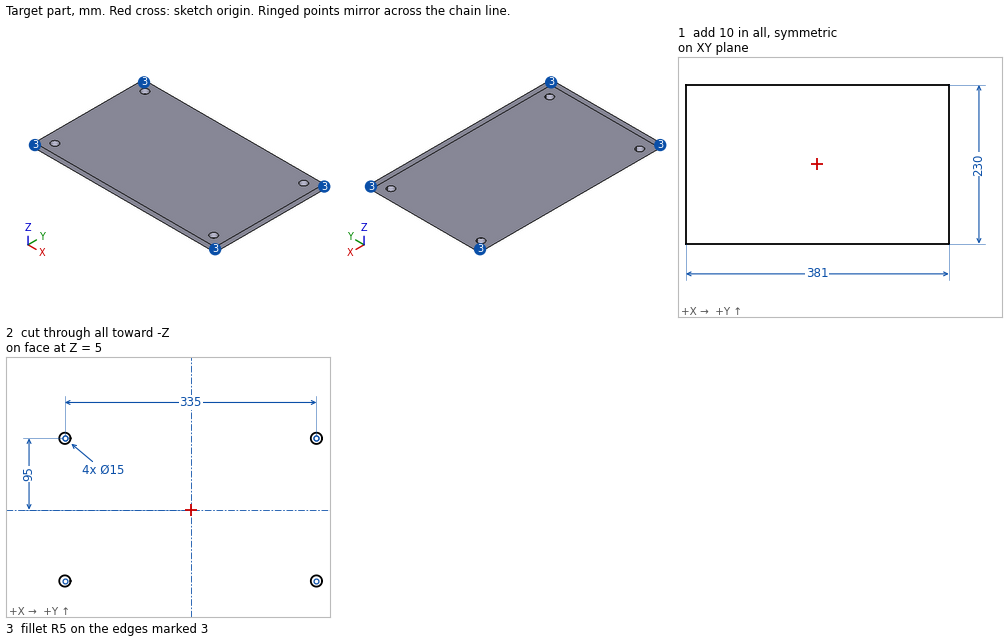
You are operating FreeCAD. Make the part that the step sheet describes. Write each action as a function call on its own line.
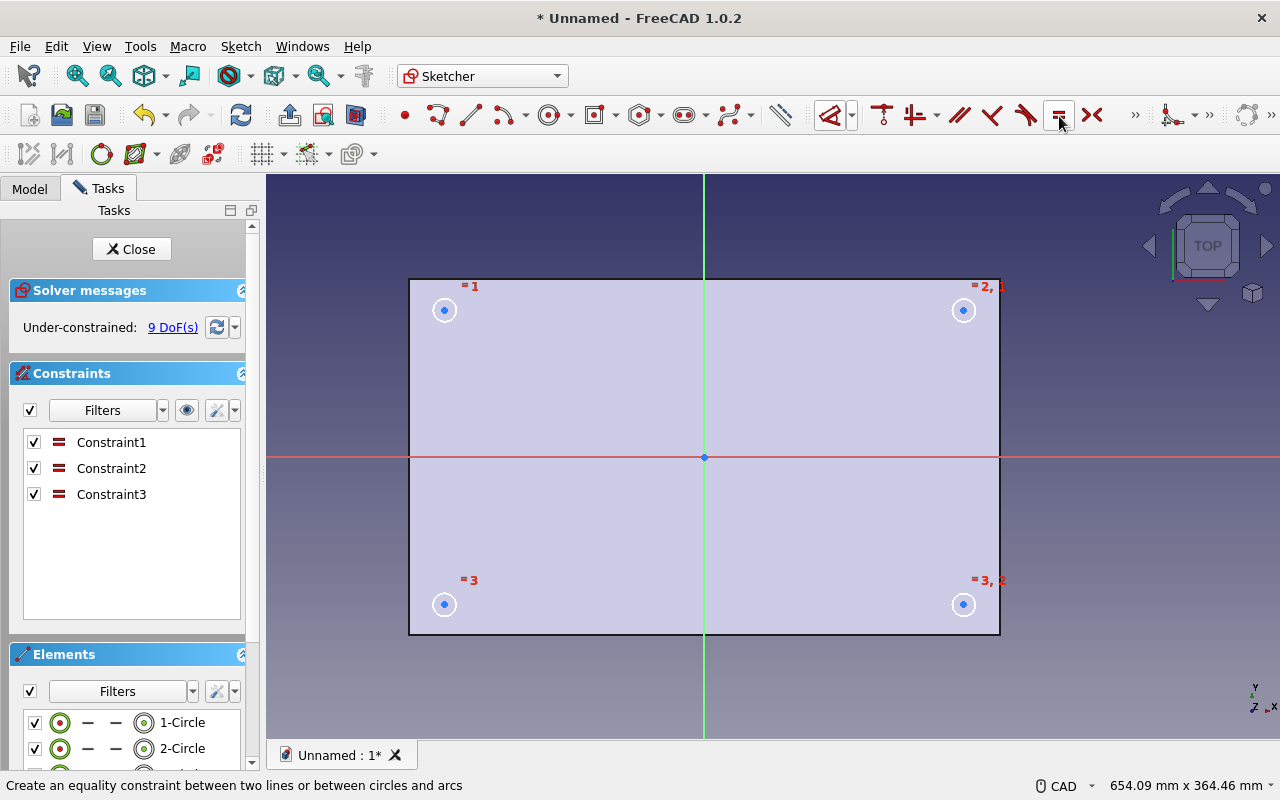
click(445, 310)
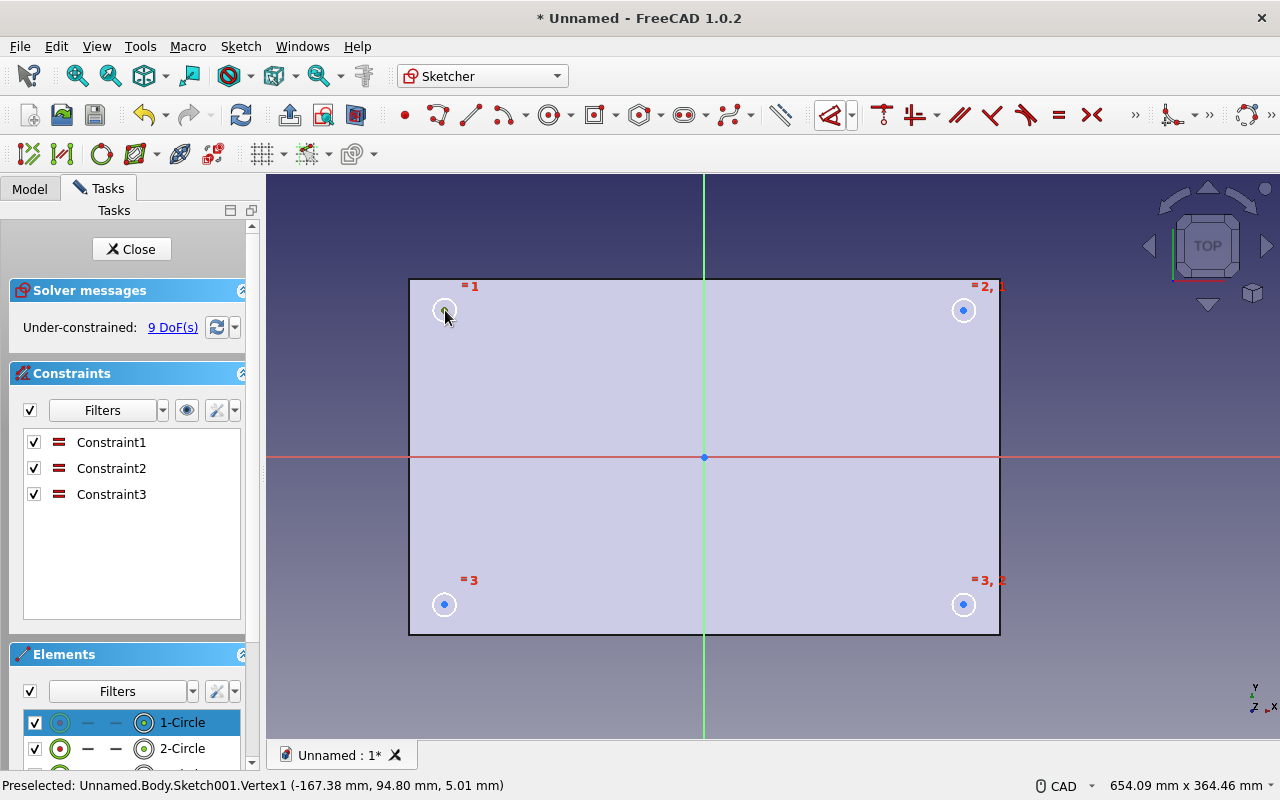
click(964, 311)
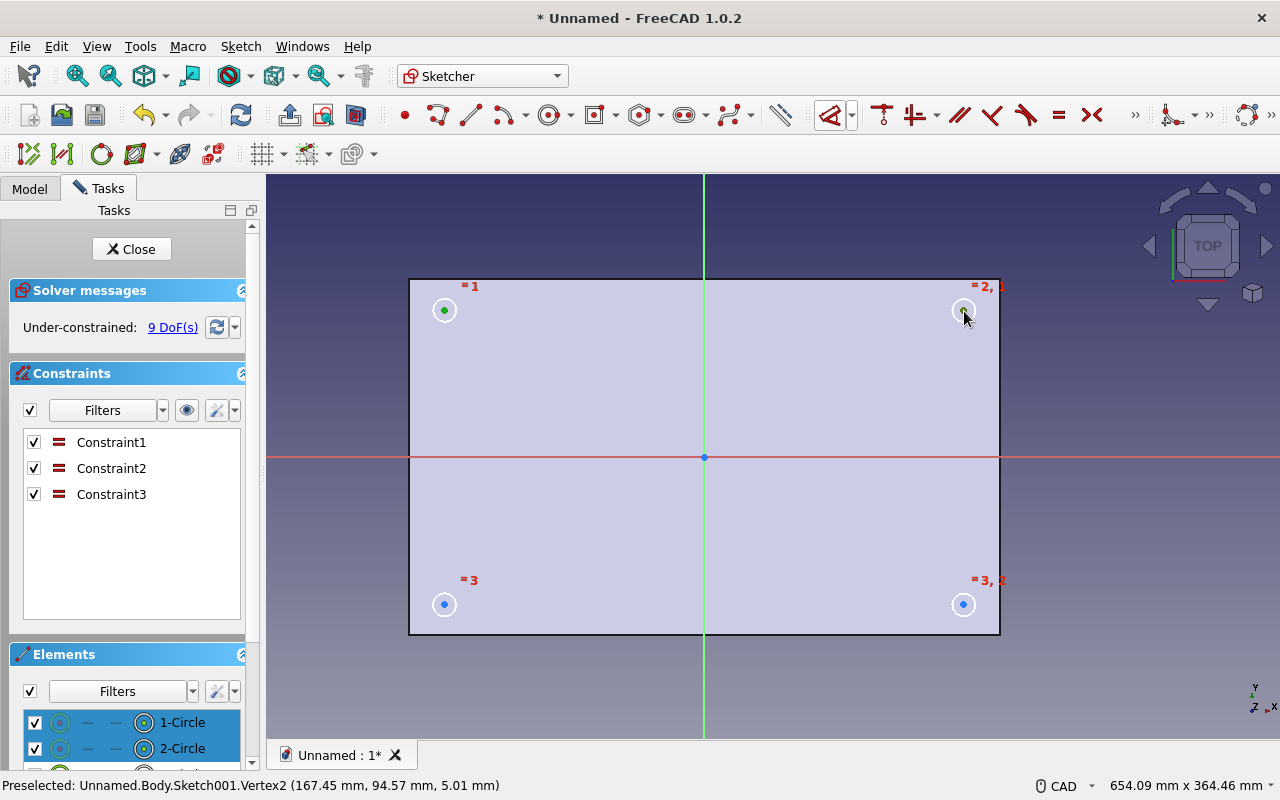
click(704, 675)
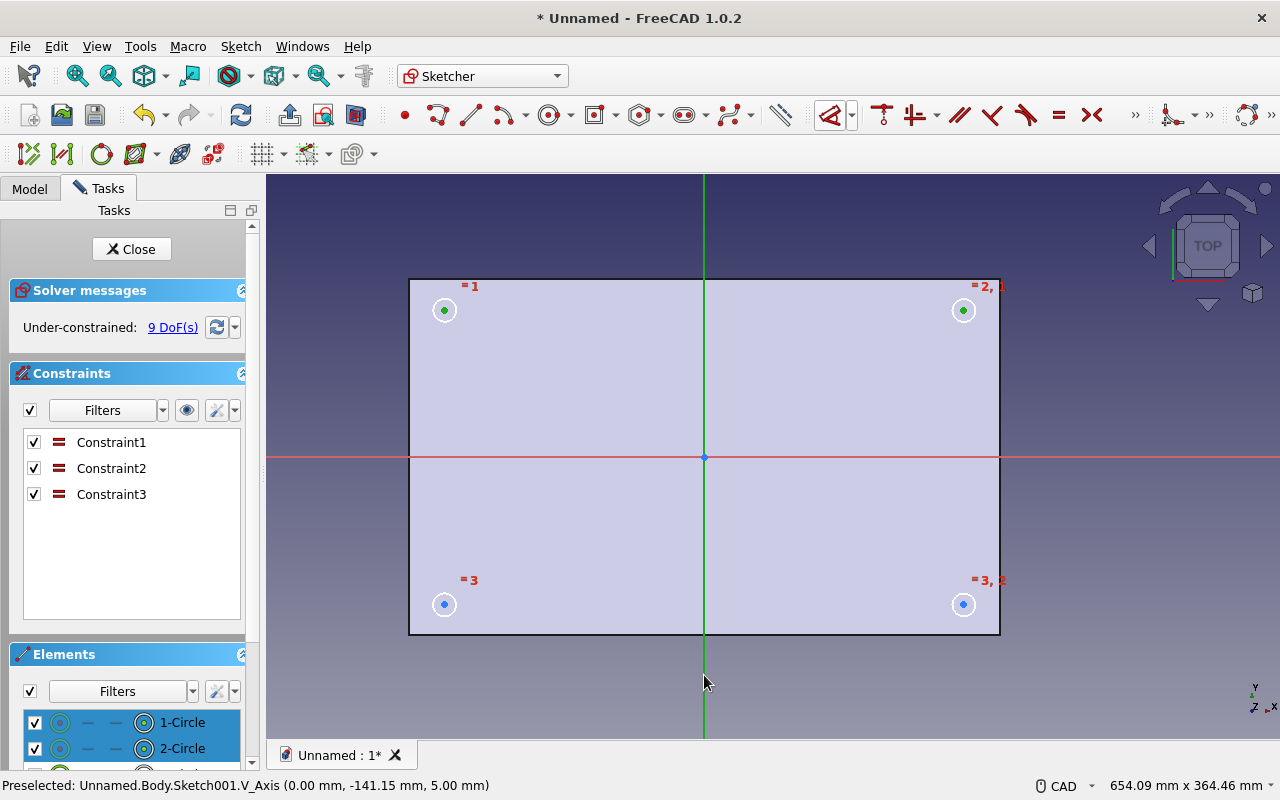
click(1092, 116)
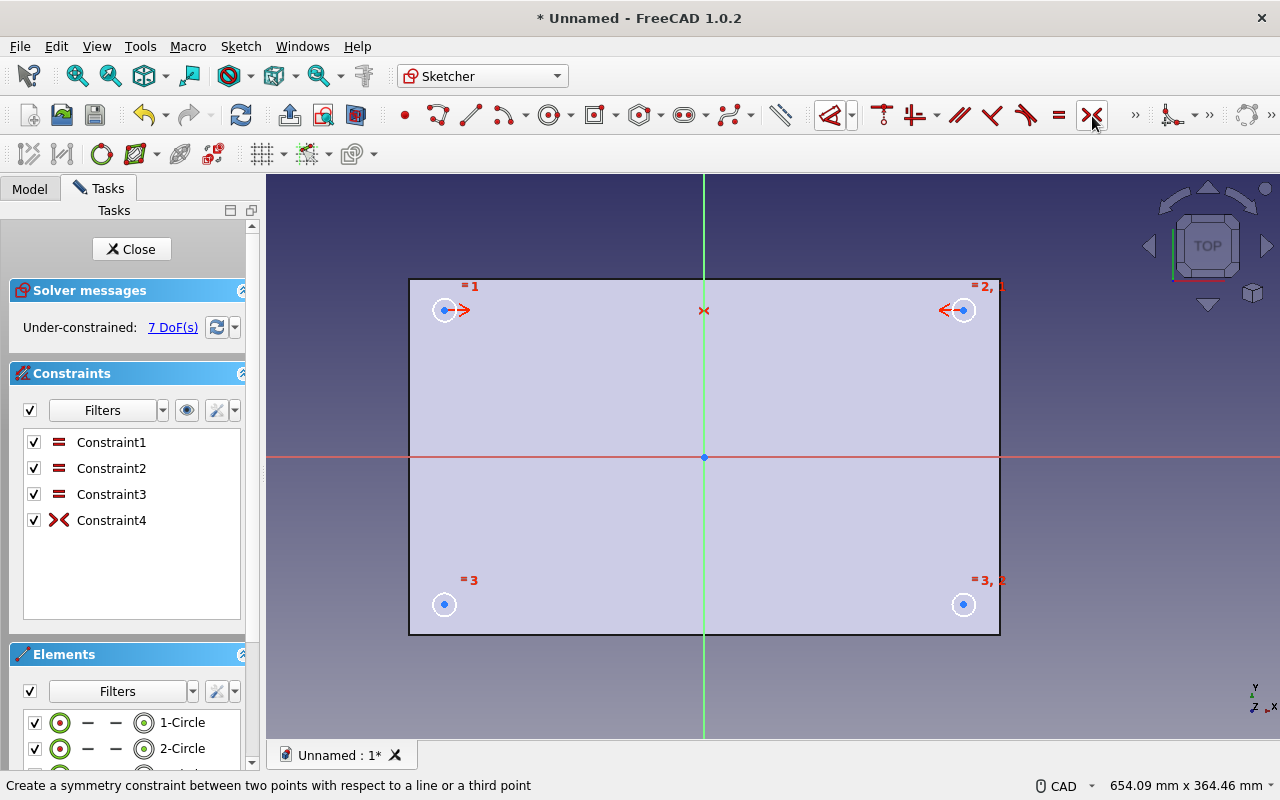
click(964, 310)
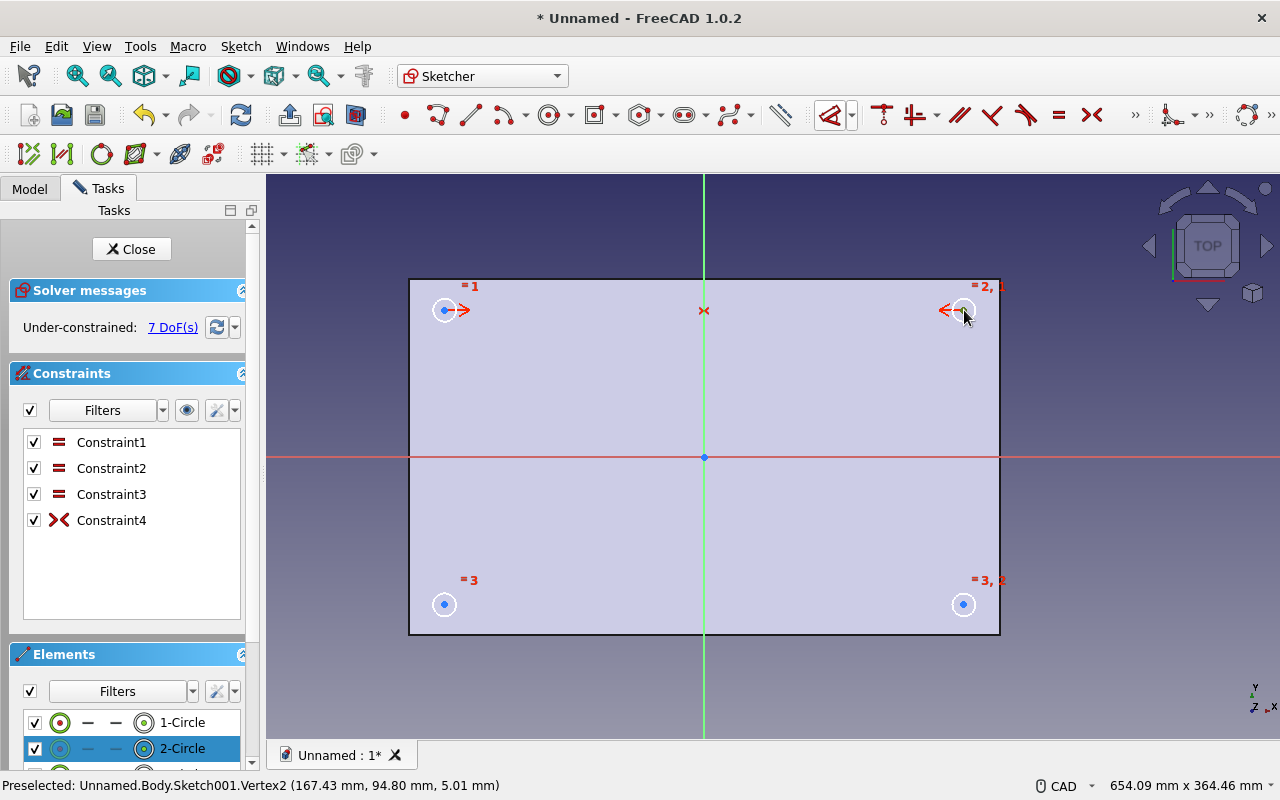
click(964, 605)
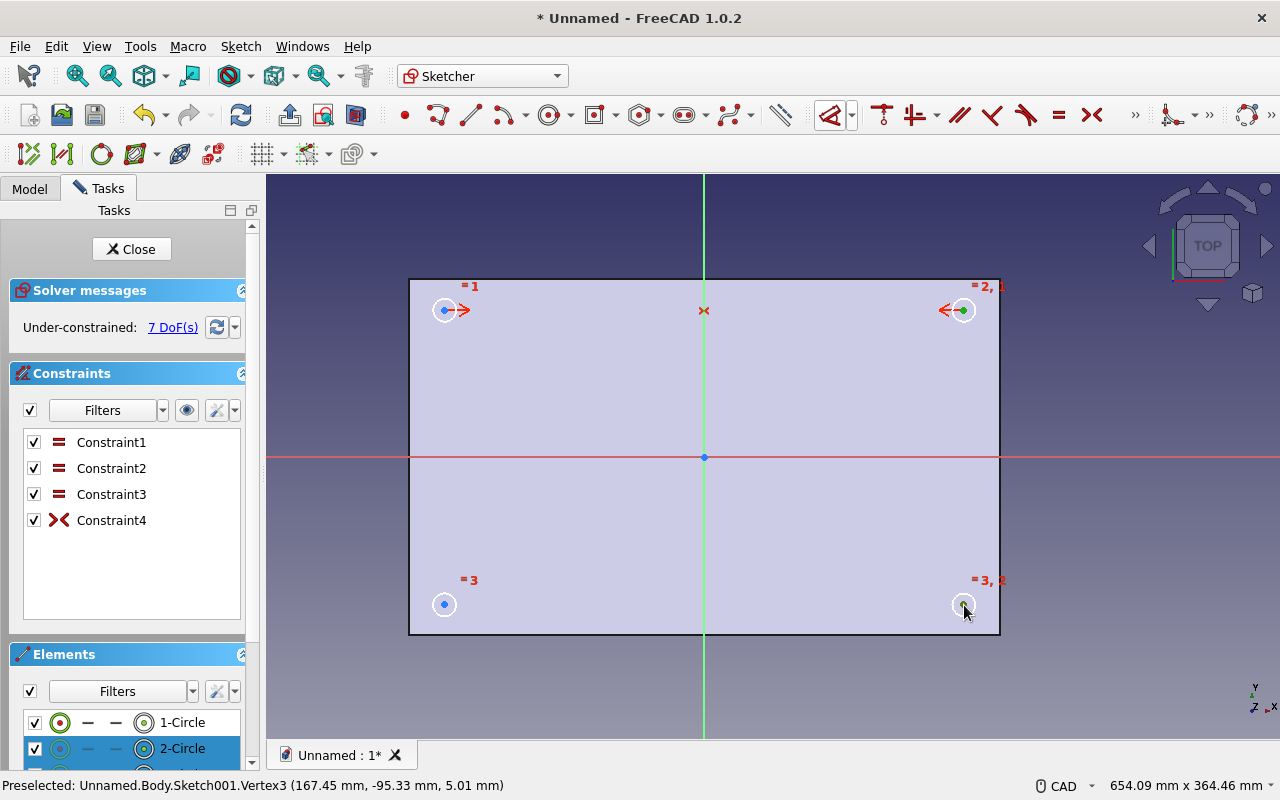
click(353, 457)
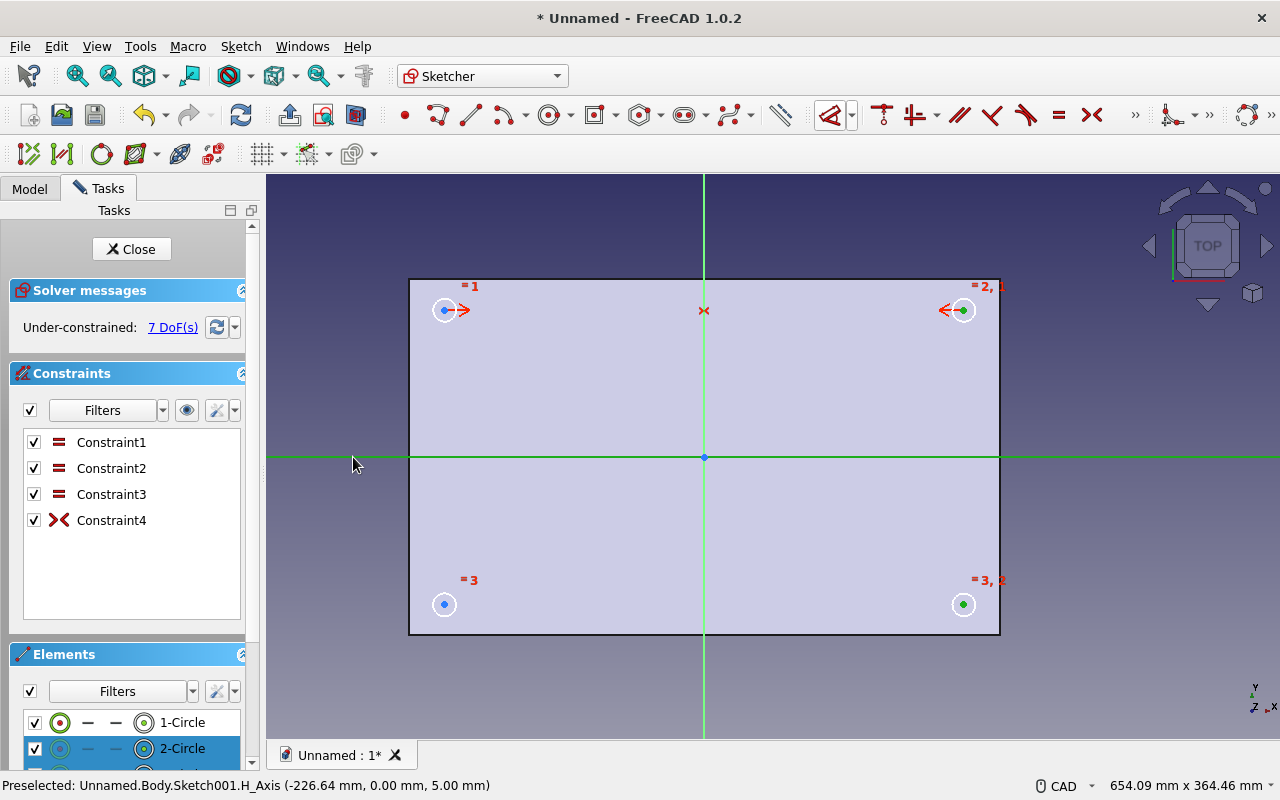
click(1092, 116)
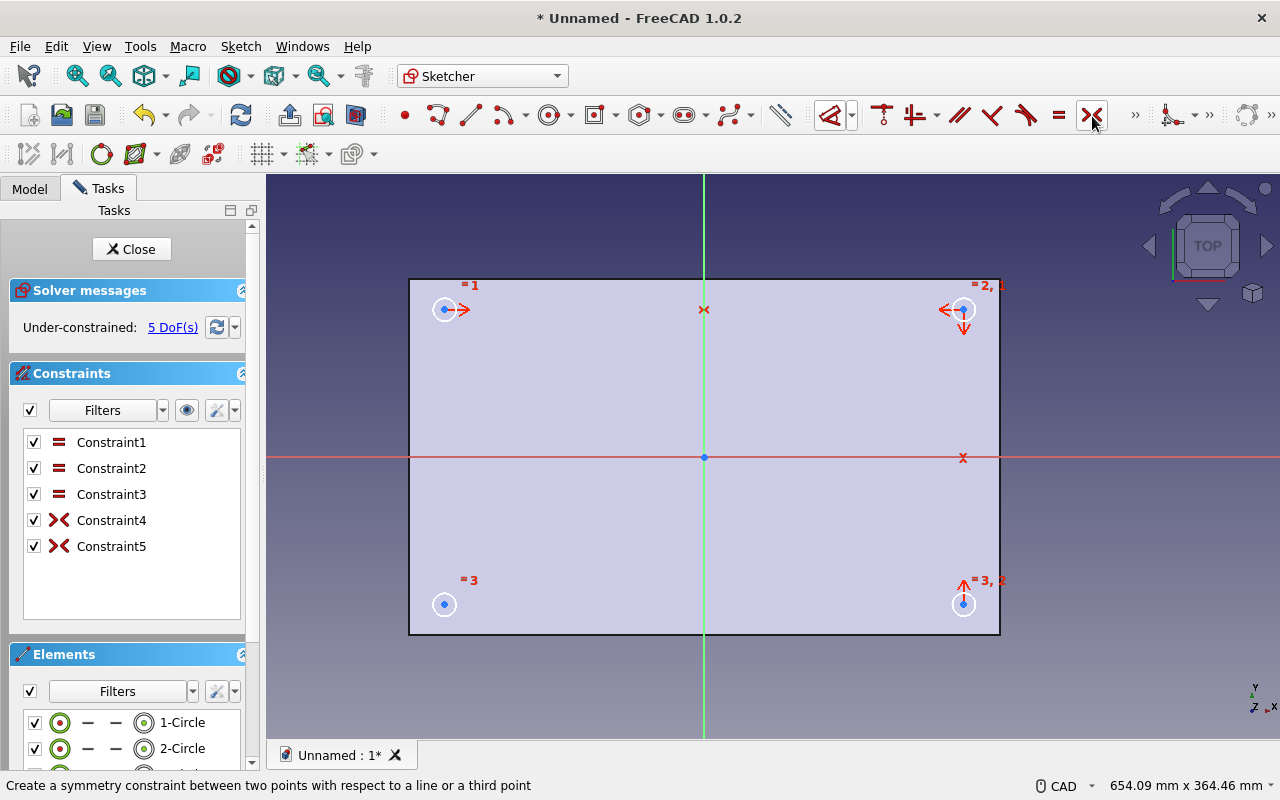
click(445, 310)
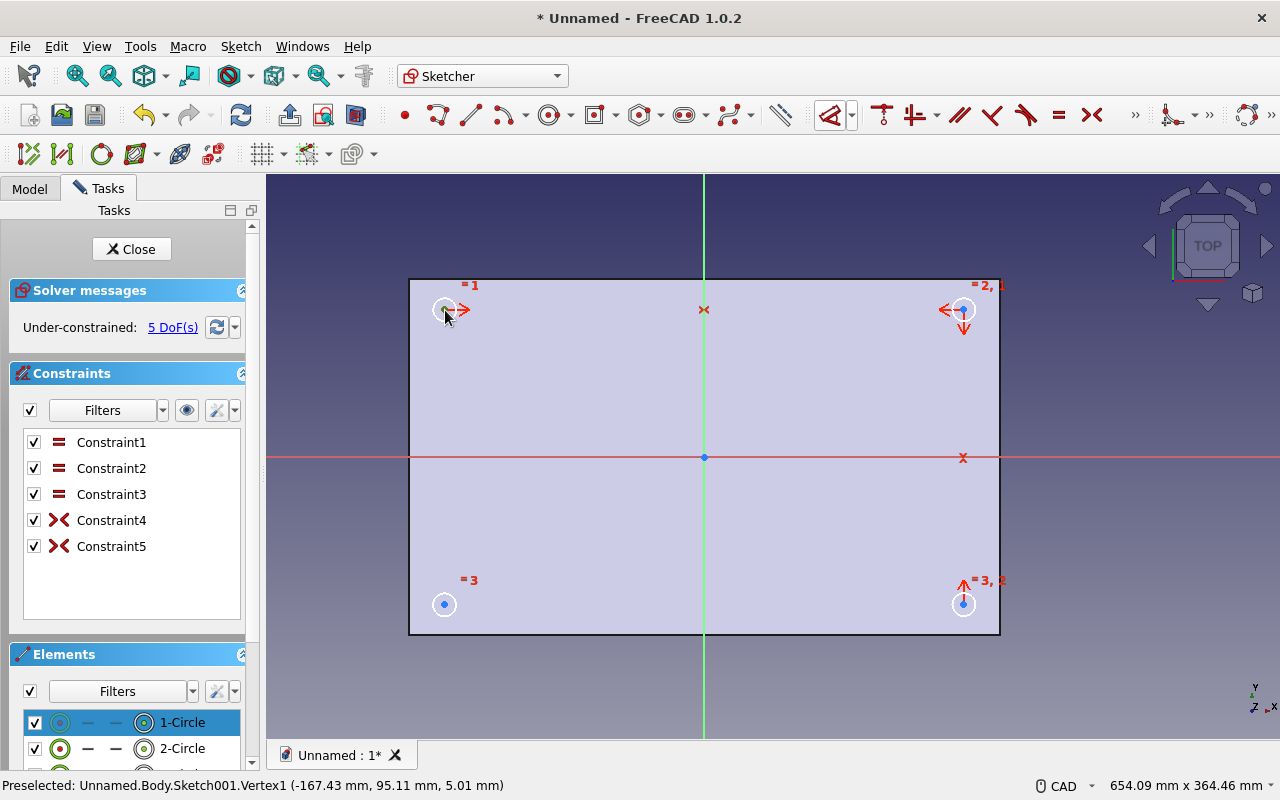
click(445, 605)